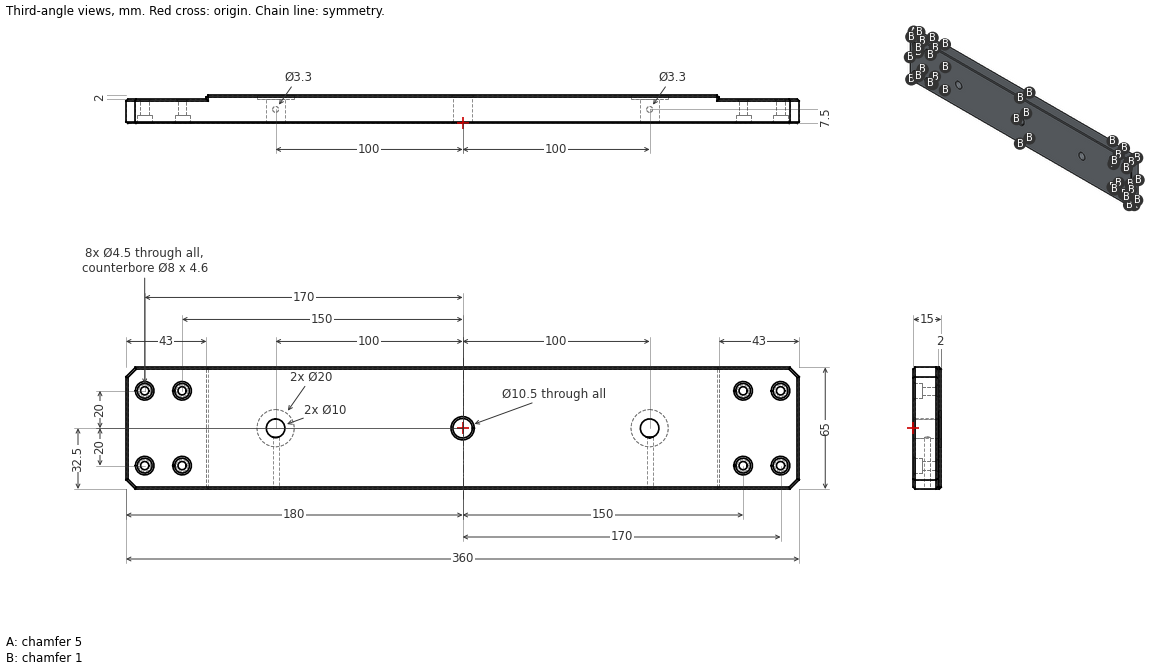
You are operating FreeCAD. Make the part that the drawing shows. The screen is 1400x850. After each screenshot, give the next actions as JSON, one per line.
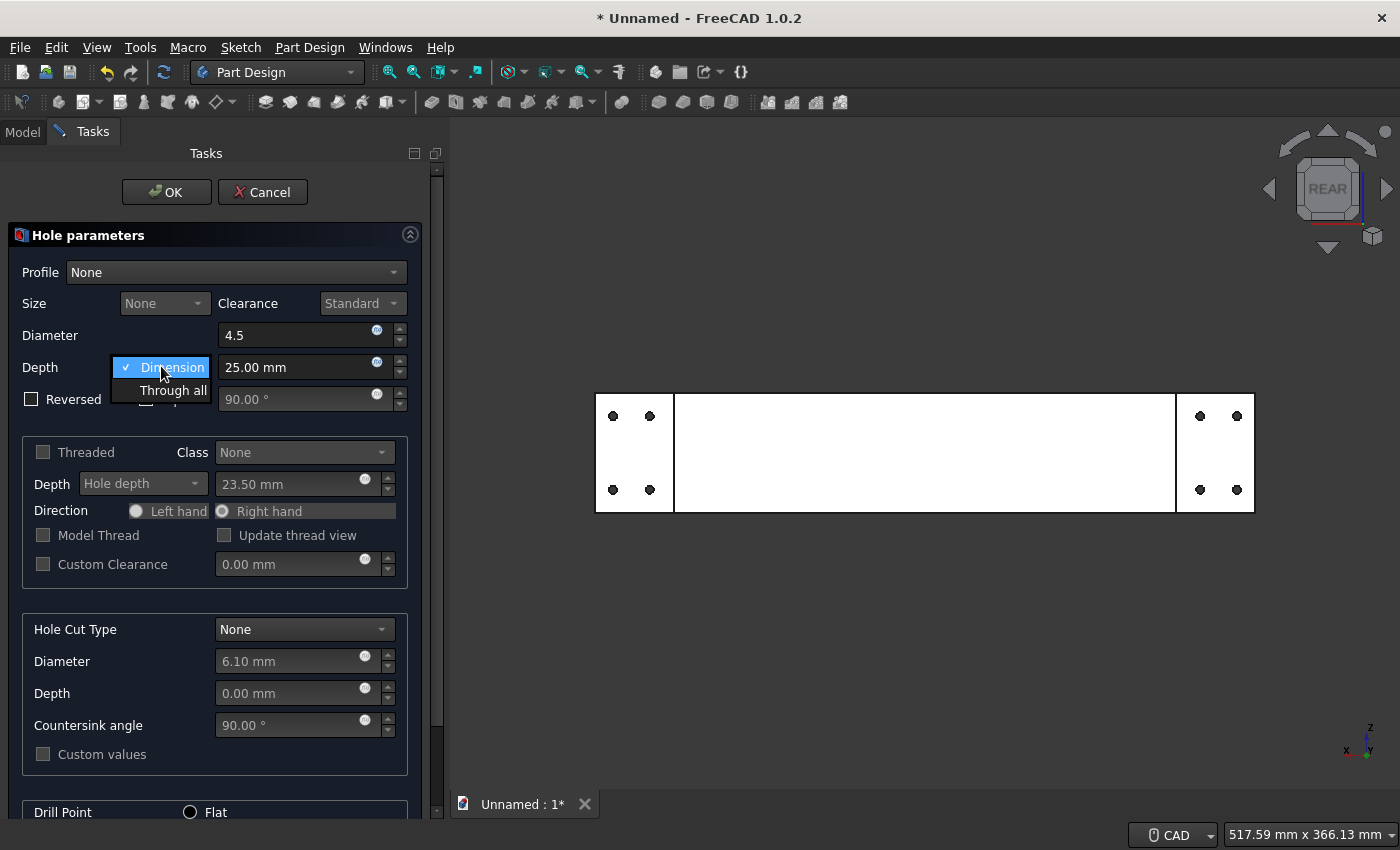
{"action": "left_click", "coordinate": [160, 390]}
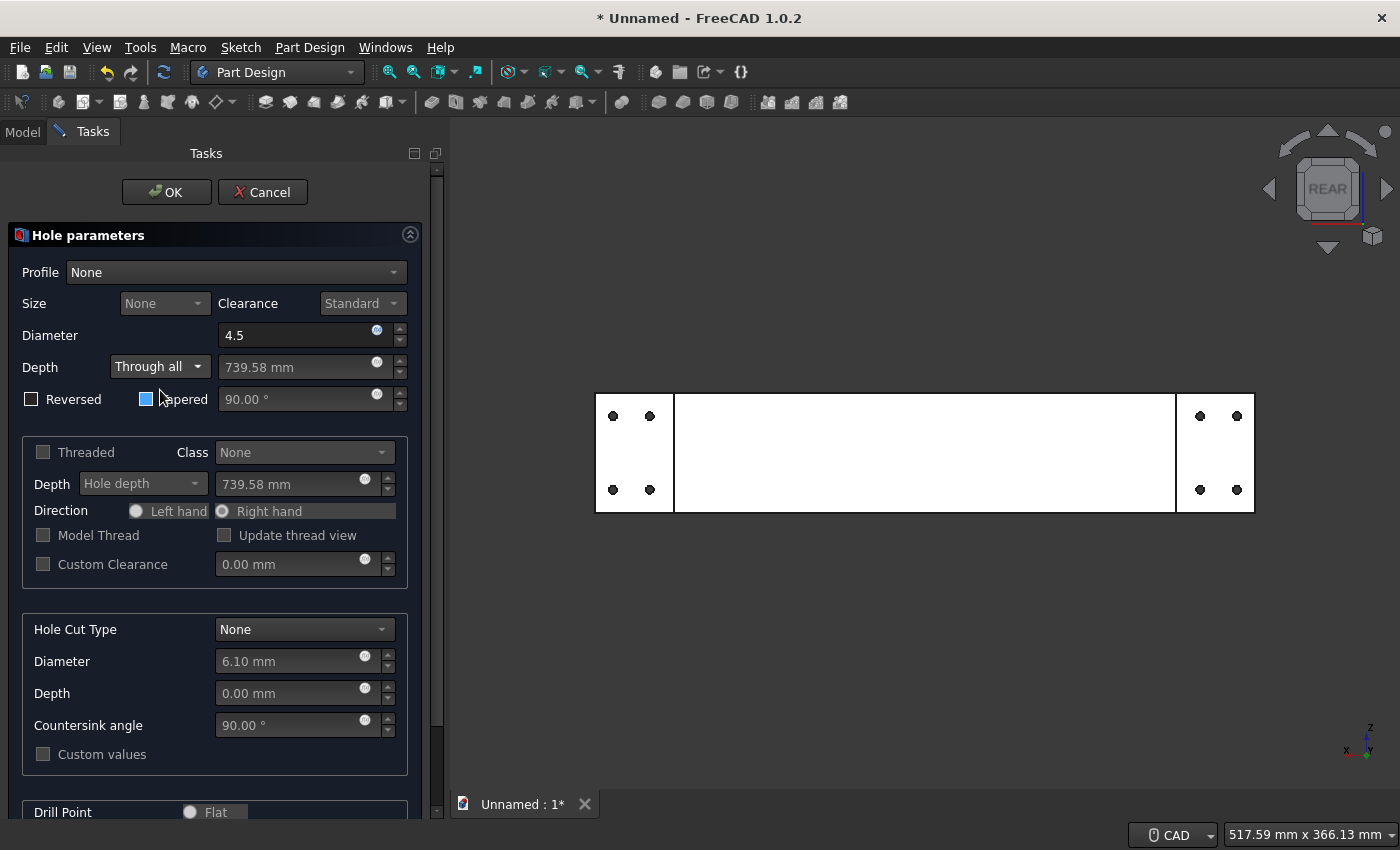
{"action": "left_click", "coordinate": [306, 630]}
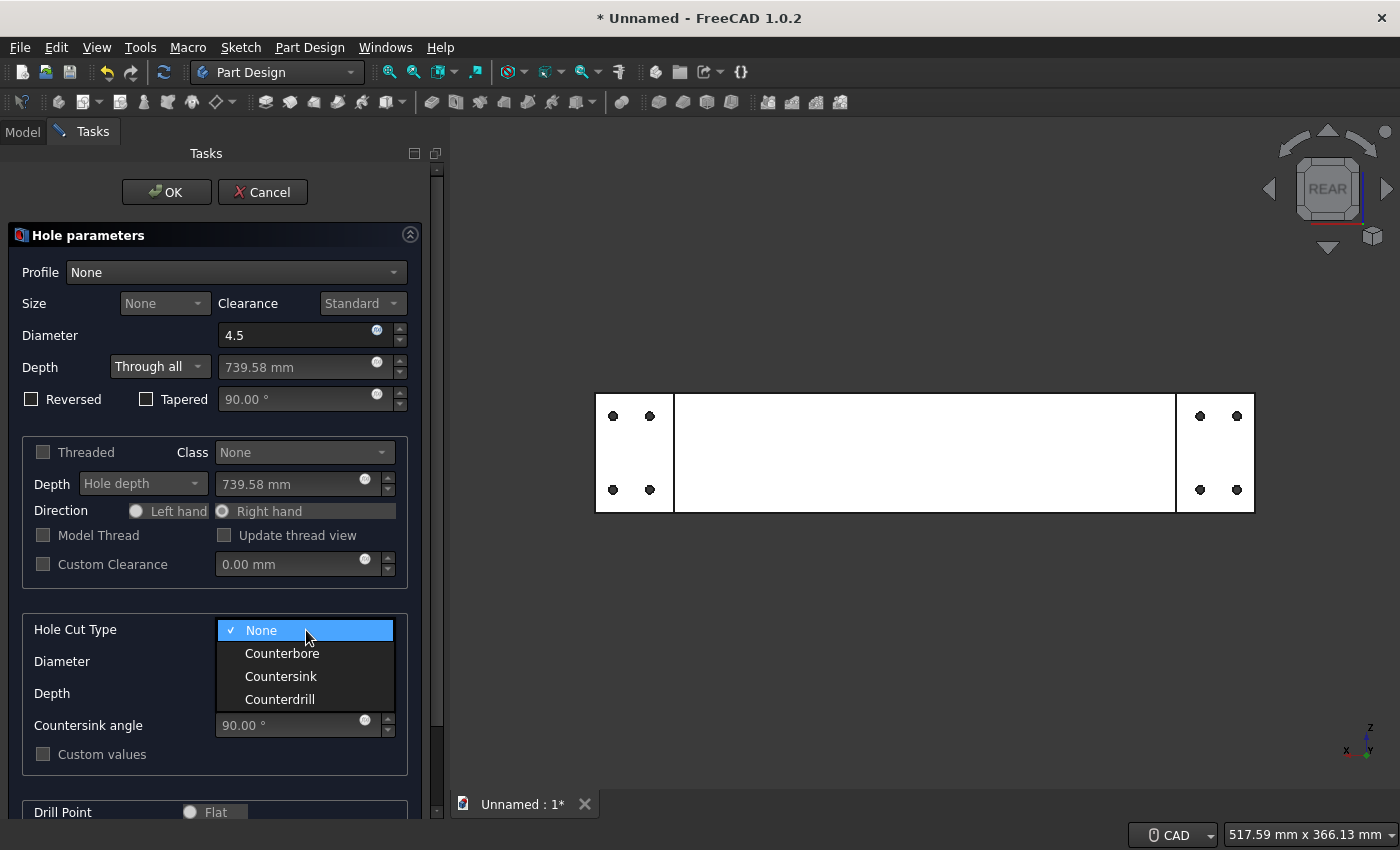
{"action": "left_click", "coordinate": [304, 654]}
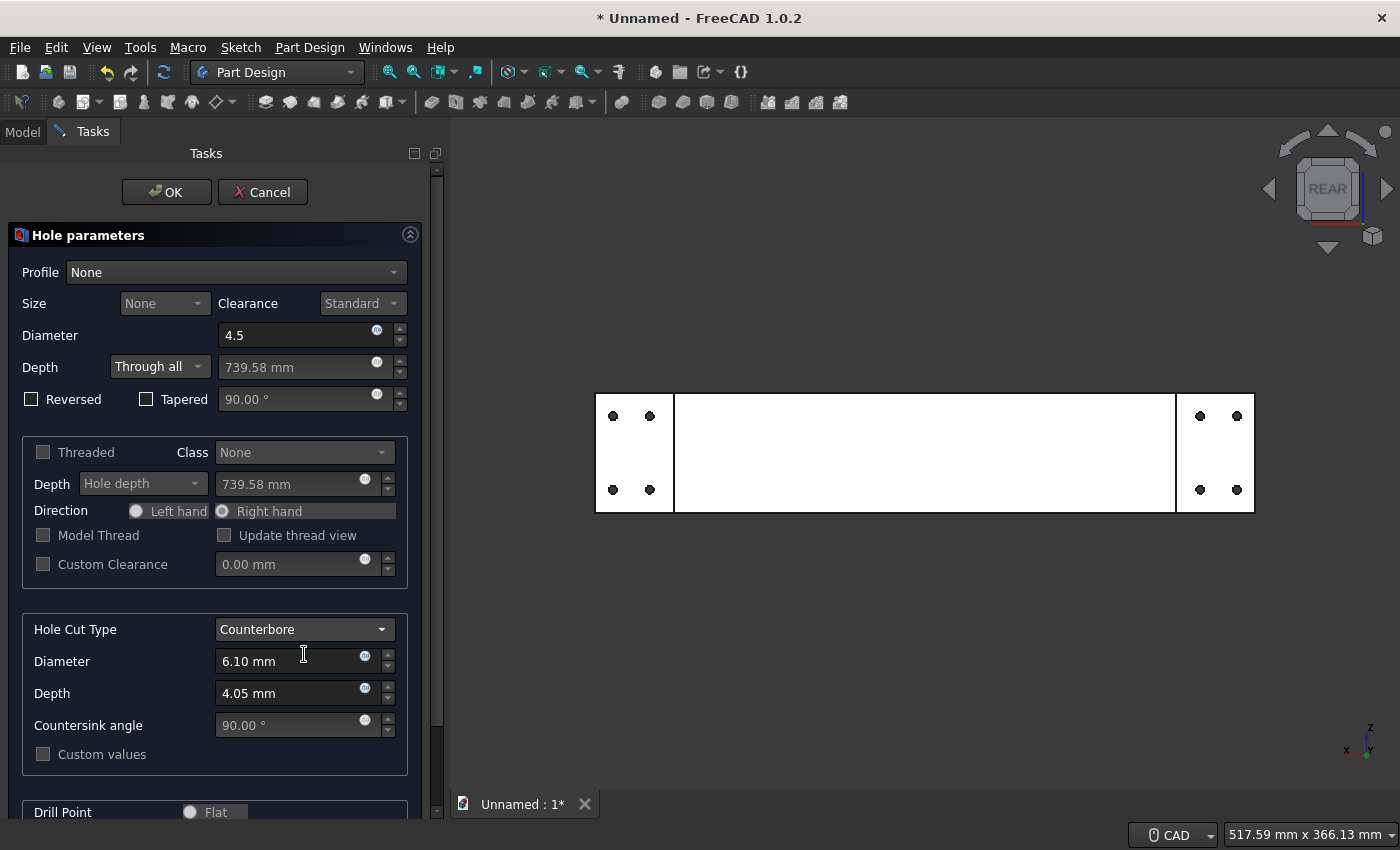
{"action": "triple_click", "coordinate": [298, 661]}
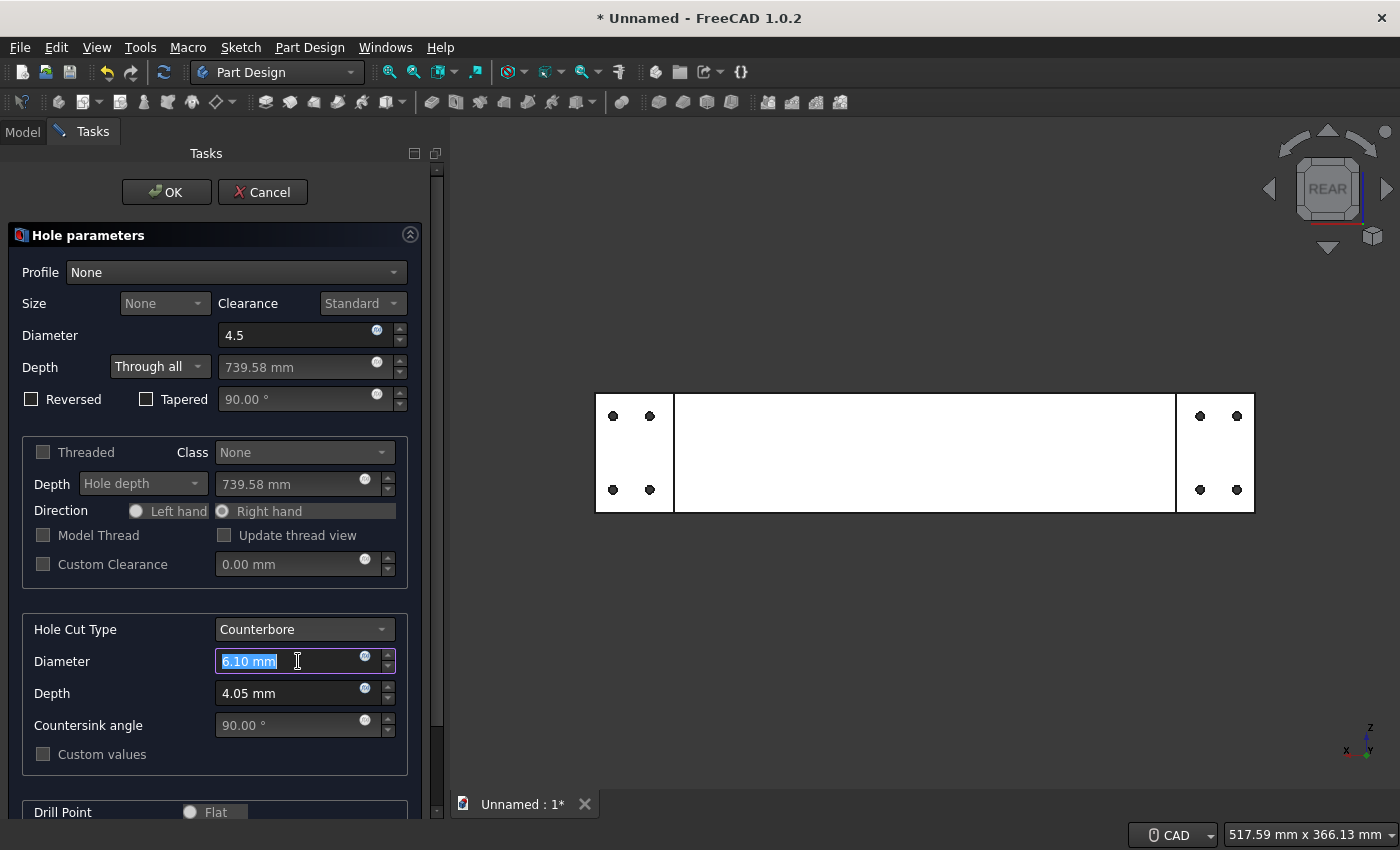
{"action": "type", "text": "8"}
{"action": "key", "text": "Tab"}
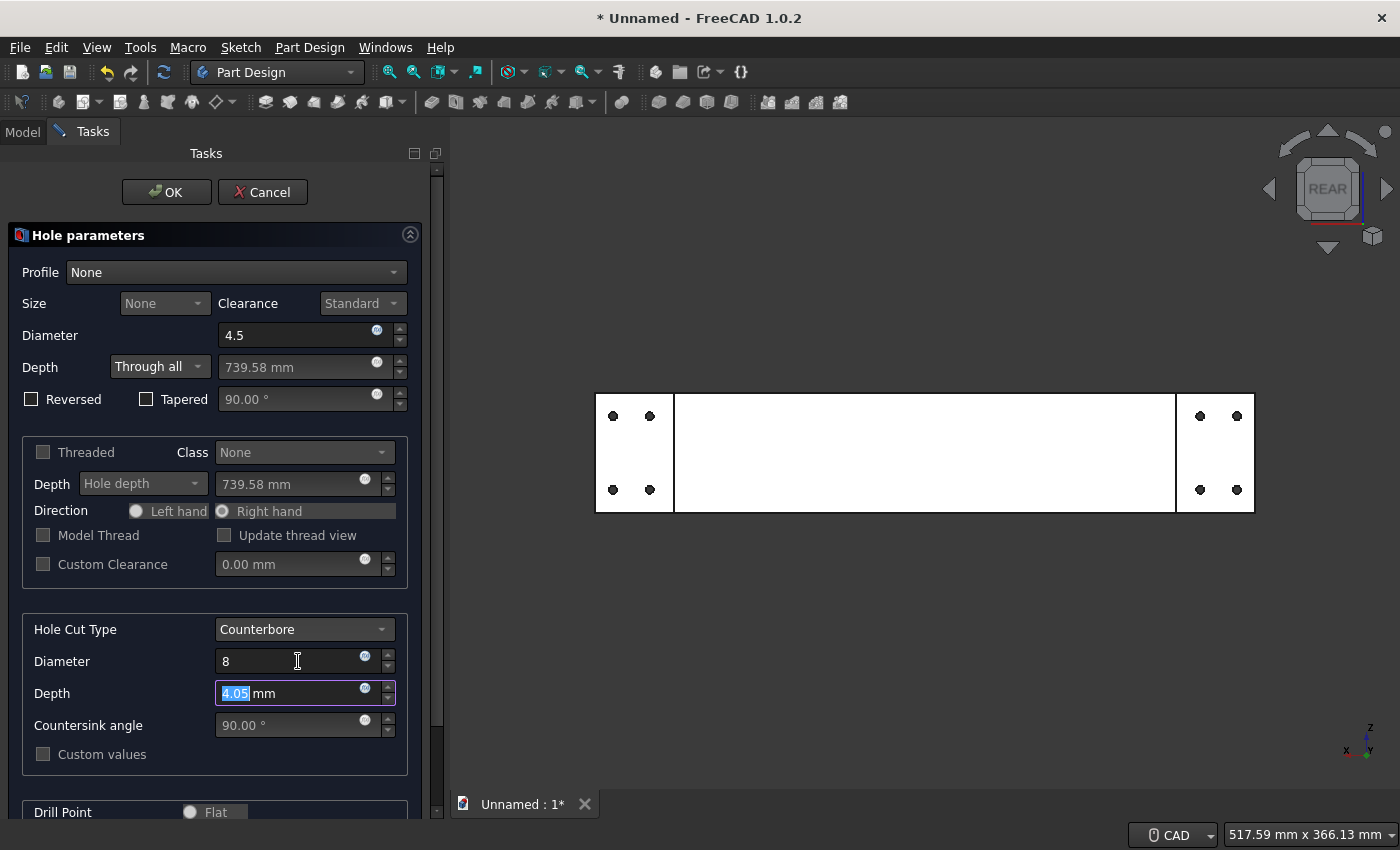
{"action": "type", "text": "4.6"}
{"action": "key", "text": "Tab"}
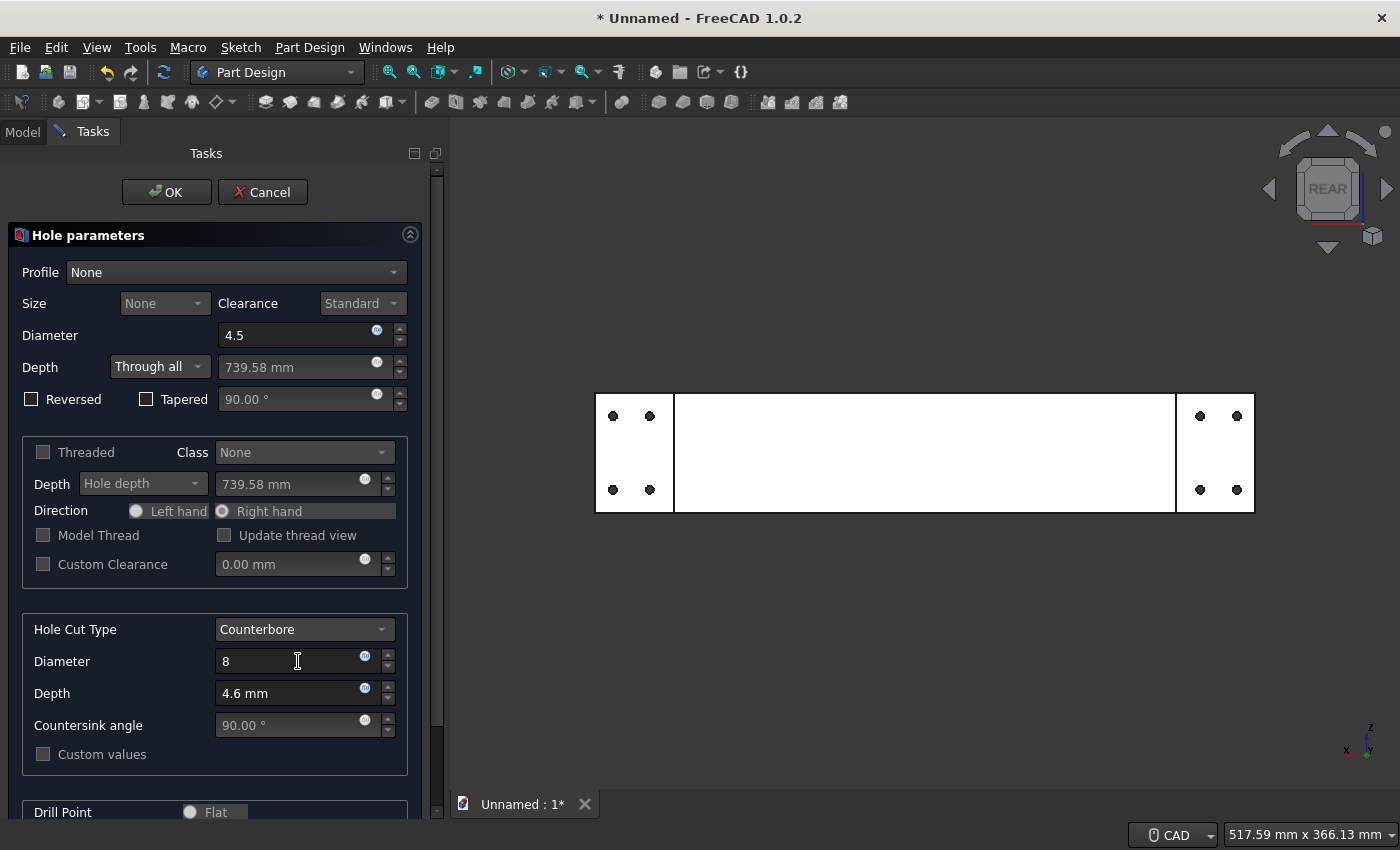
{"action": "left_click", "coordinate": [167, 192]}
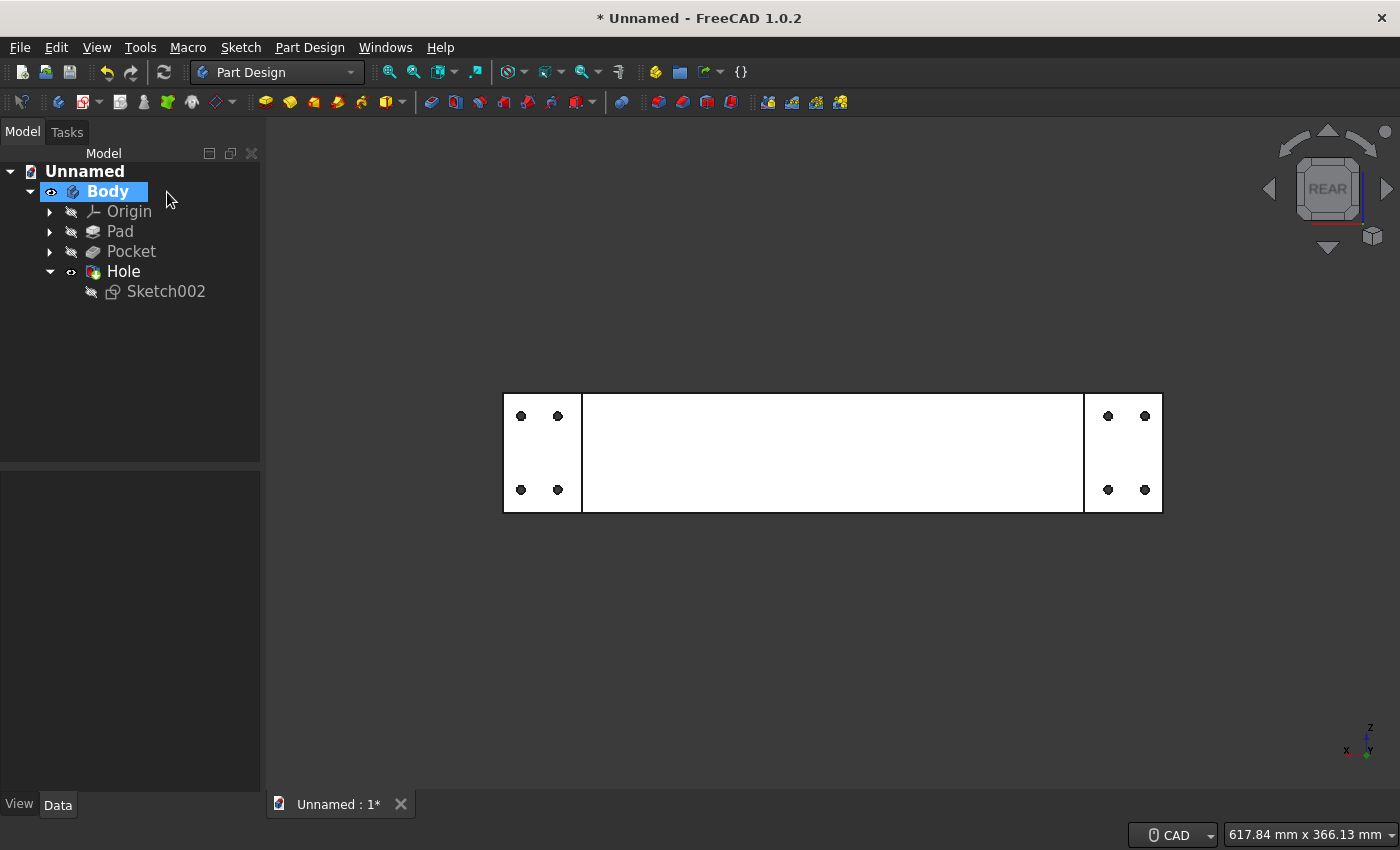
{"action": "left_click", "coordinate": [84, 102]}